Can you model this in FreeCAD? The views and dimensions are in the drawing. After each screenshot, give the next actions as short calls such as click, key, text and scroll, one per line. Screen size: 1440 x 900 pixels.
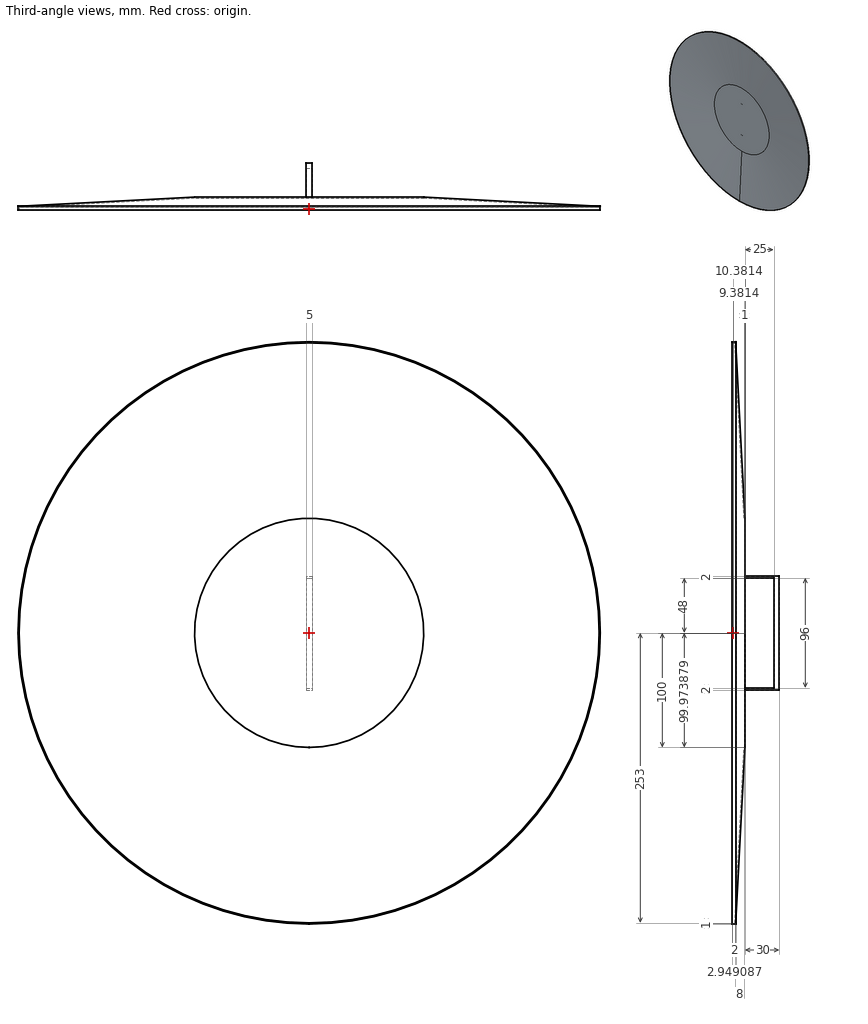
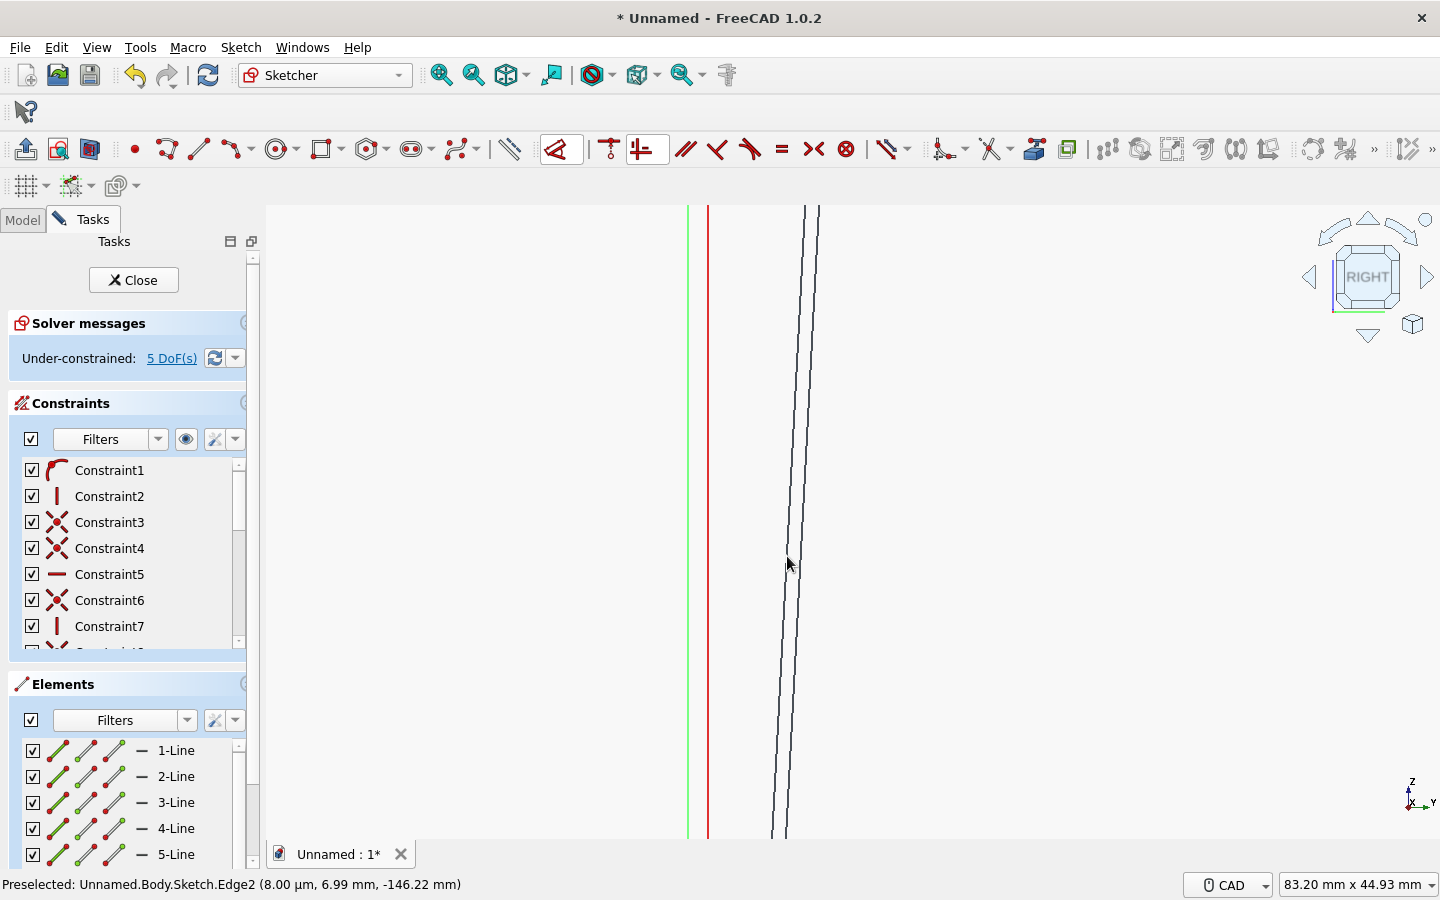
scroll(788, 551, down, 11)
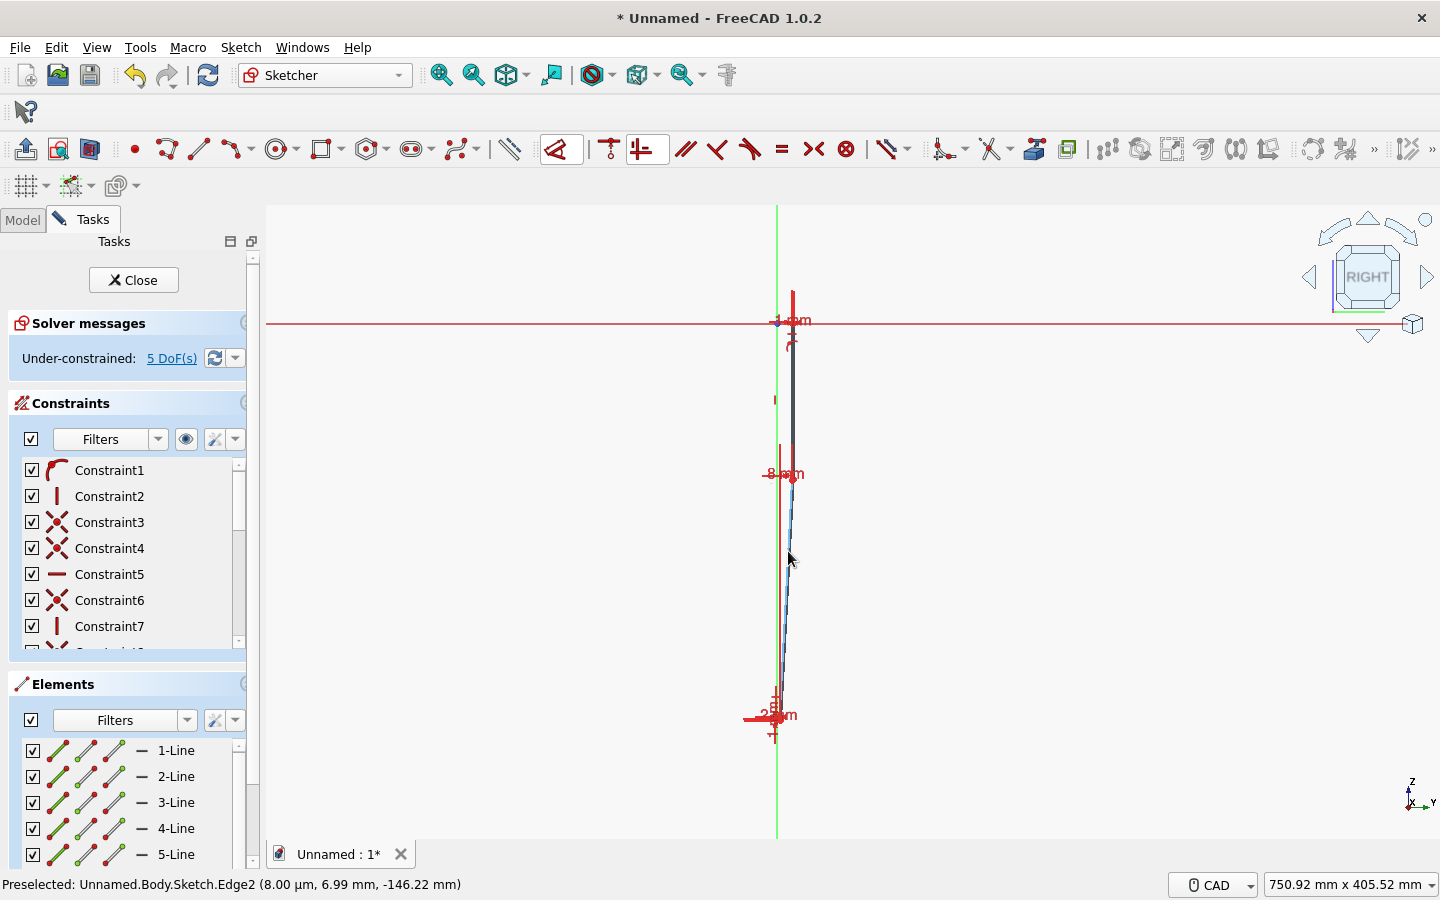
scroll(794, 433, up, 11)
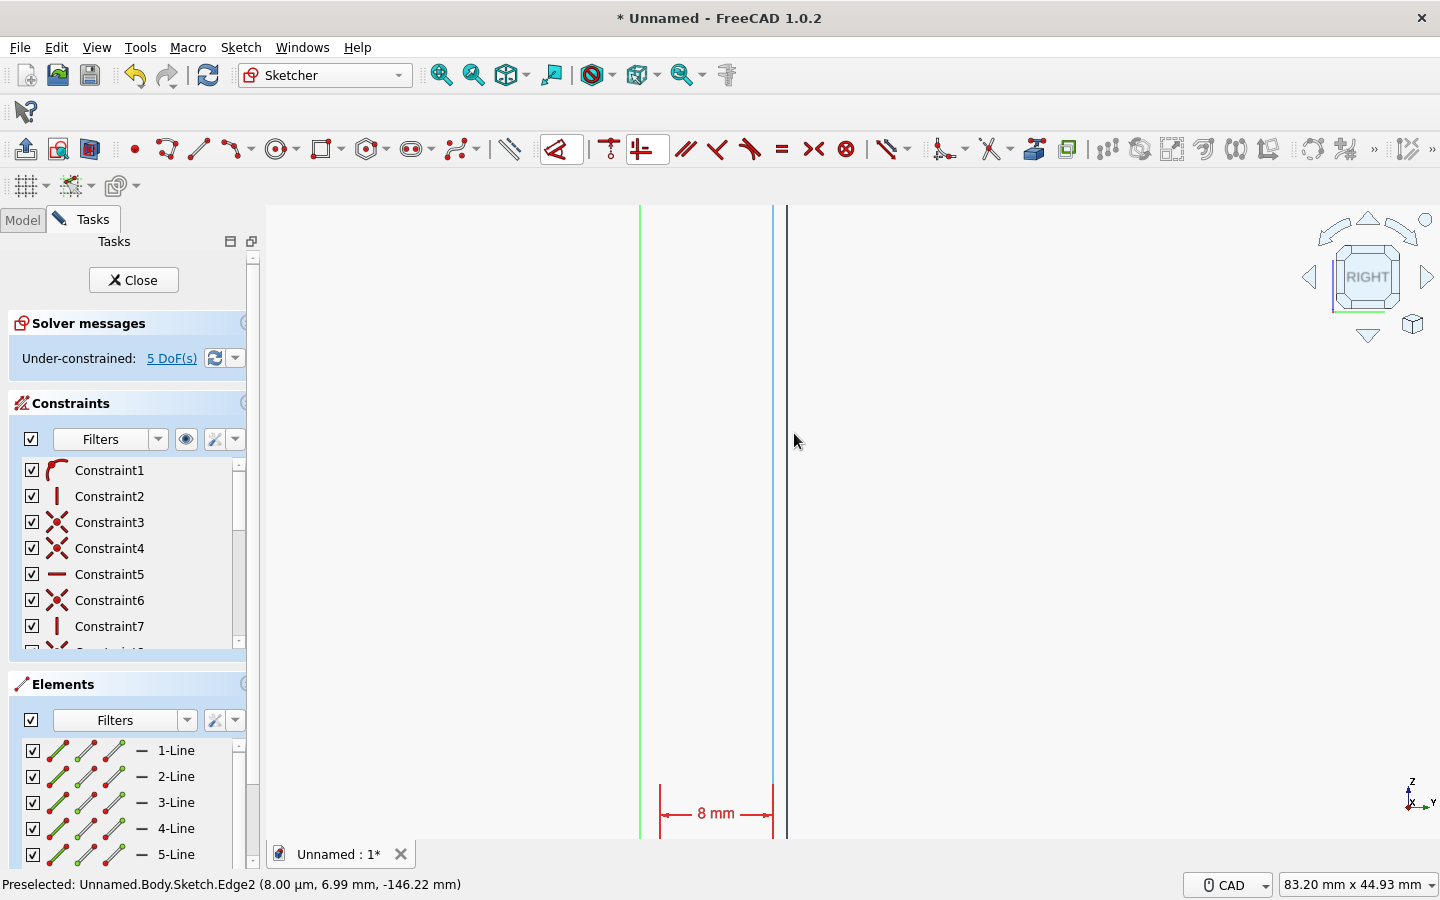
click(787, 430)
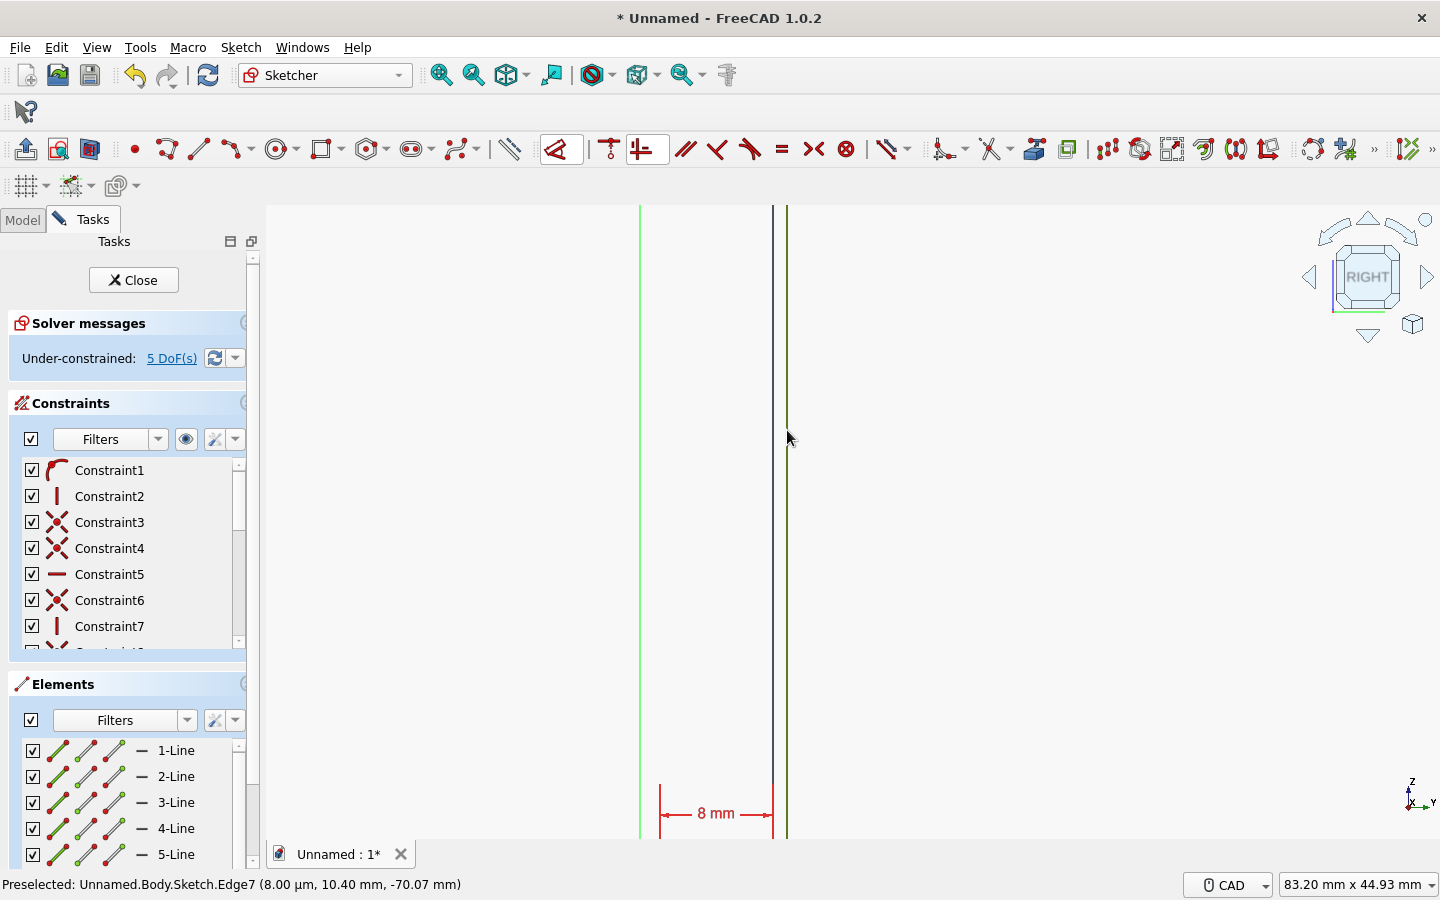
key(i)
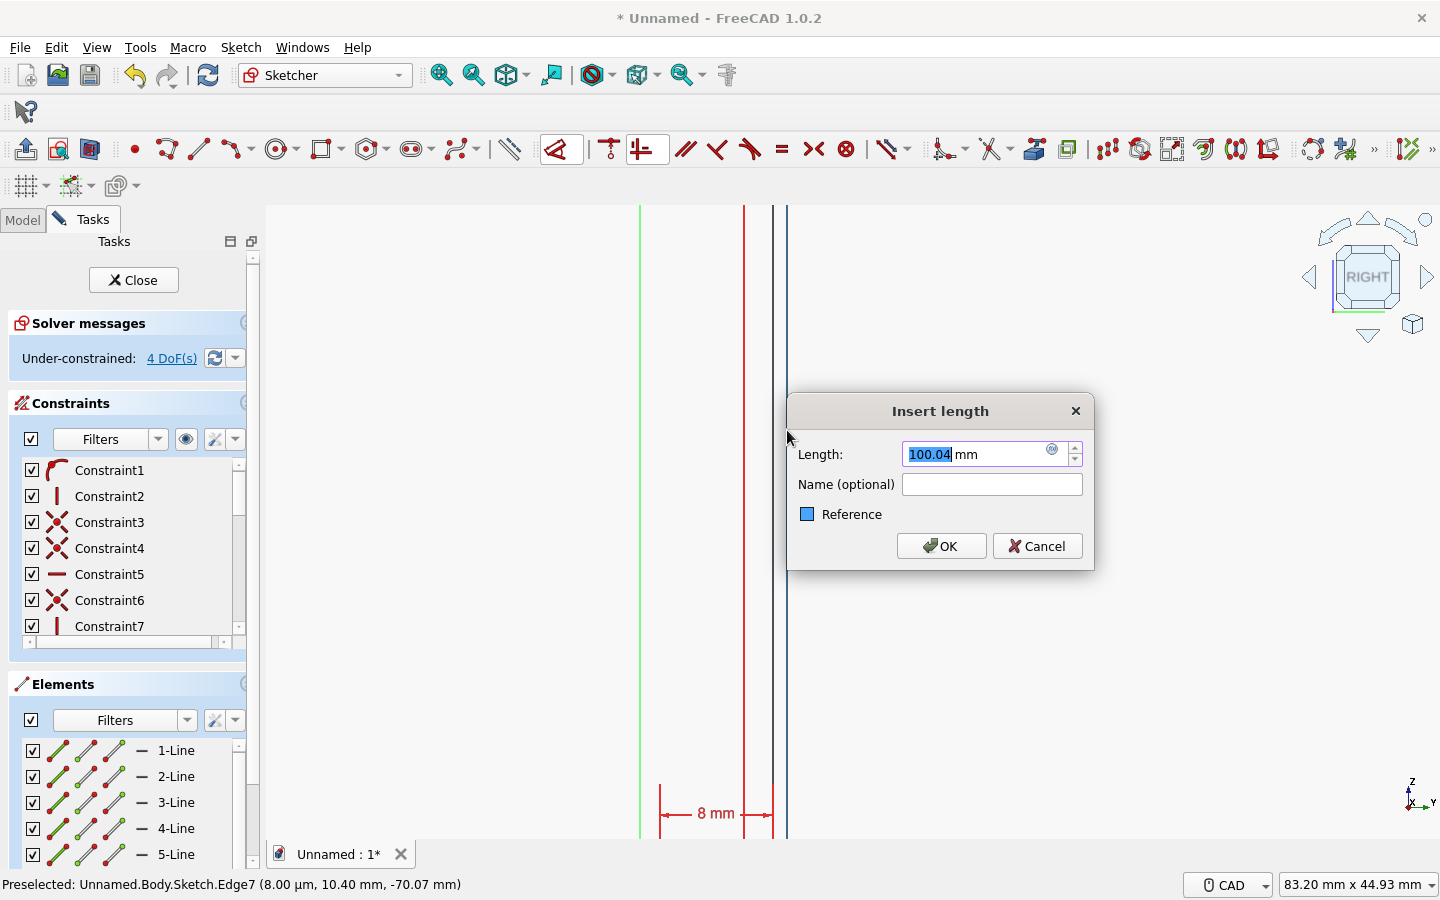
text(100)
key(Return)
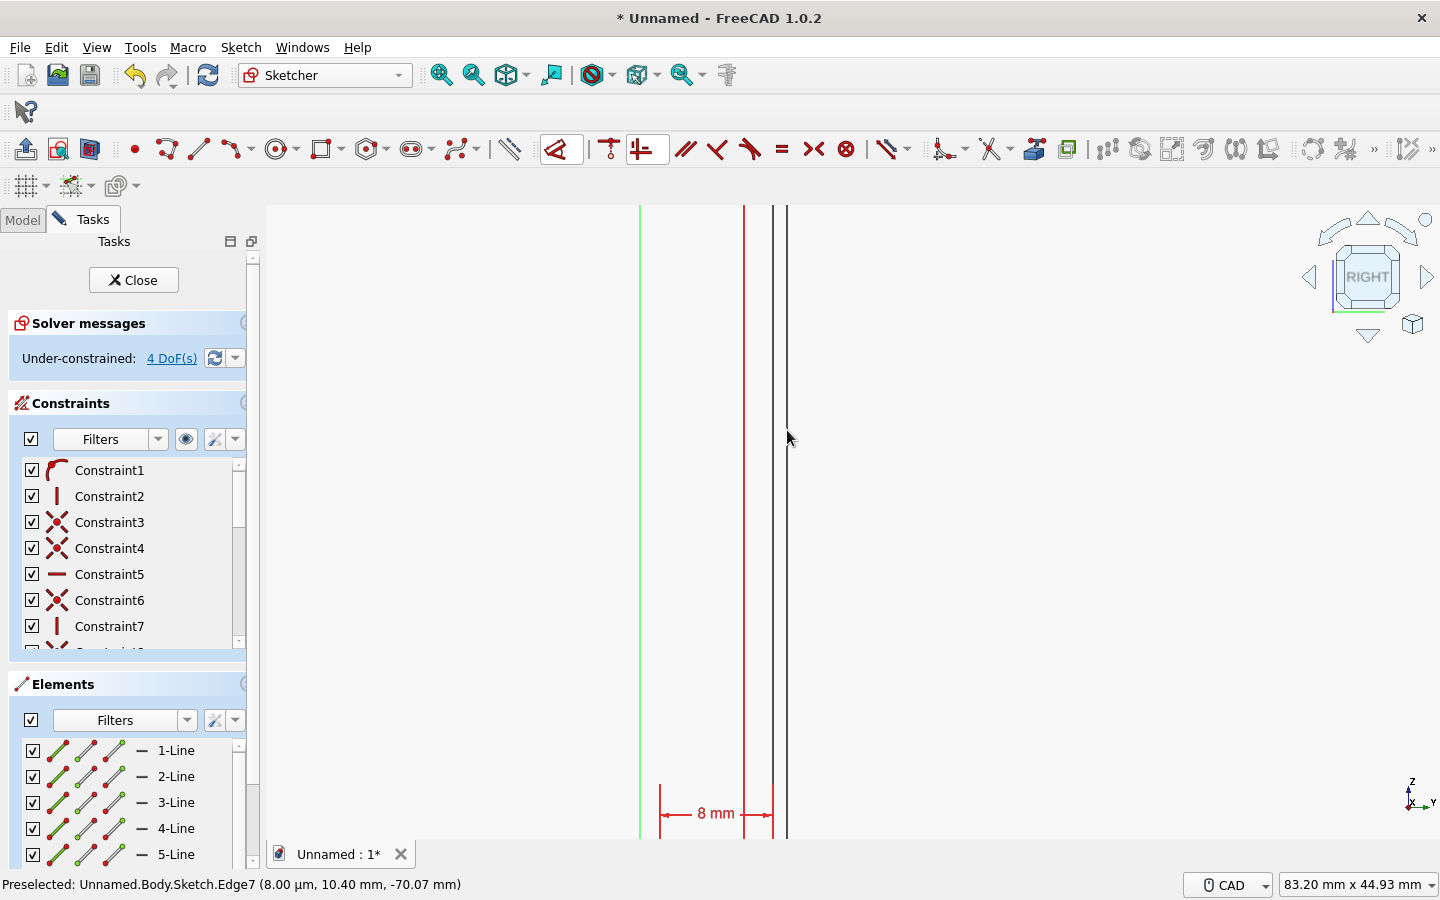
scroll(794, 433, down, 11)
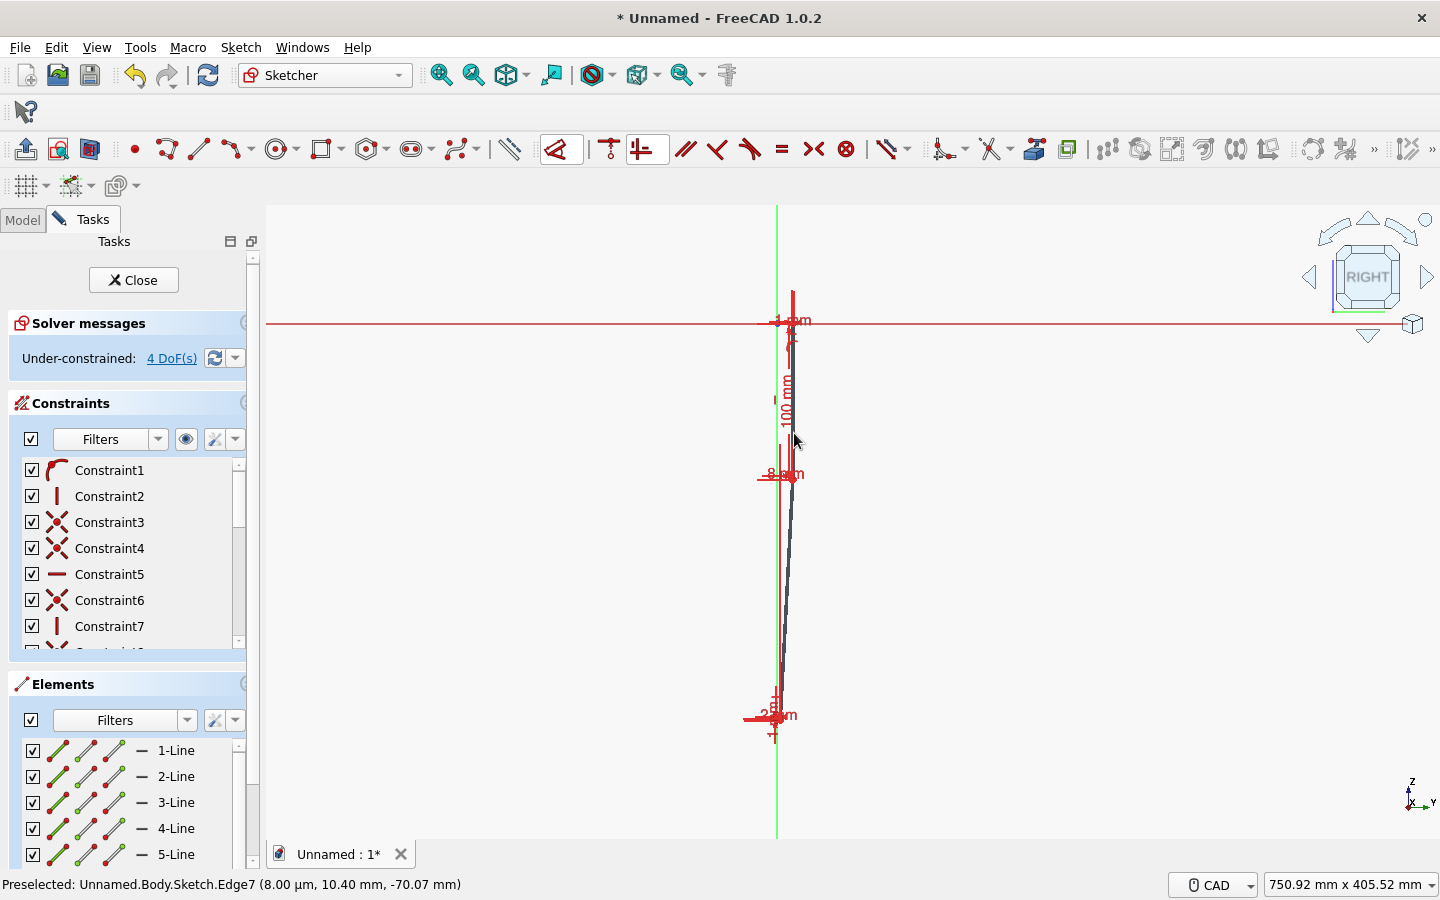
scroll(780, 719, up, 9)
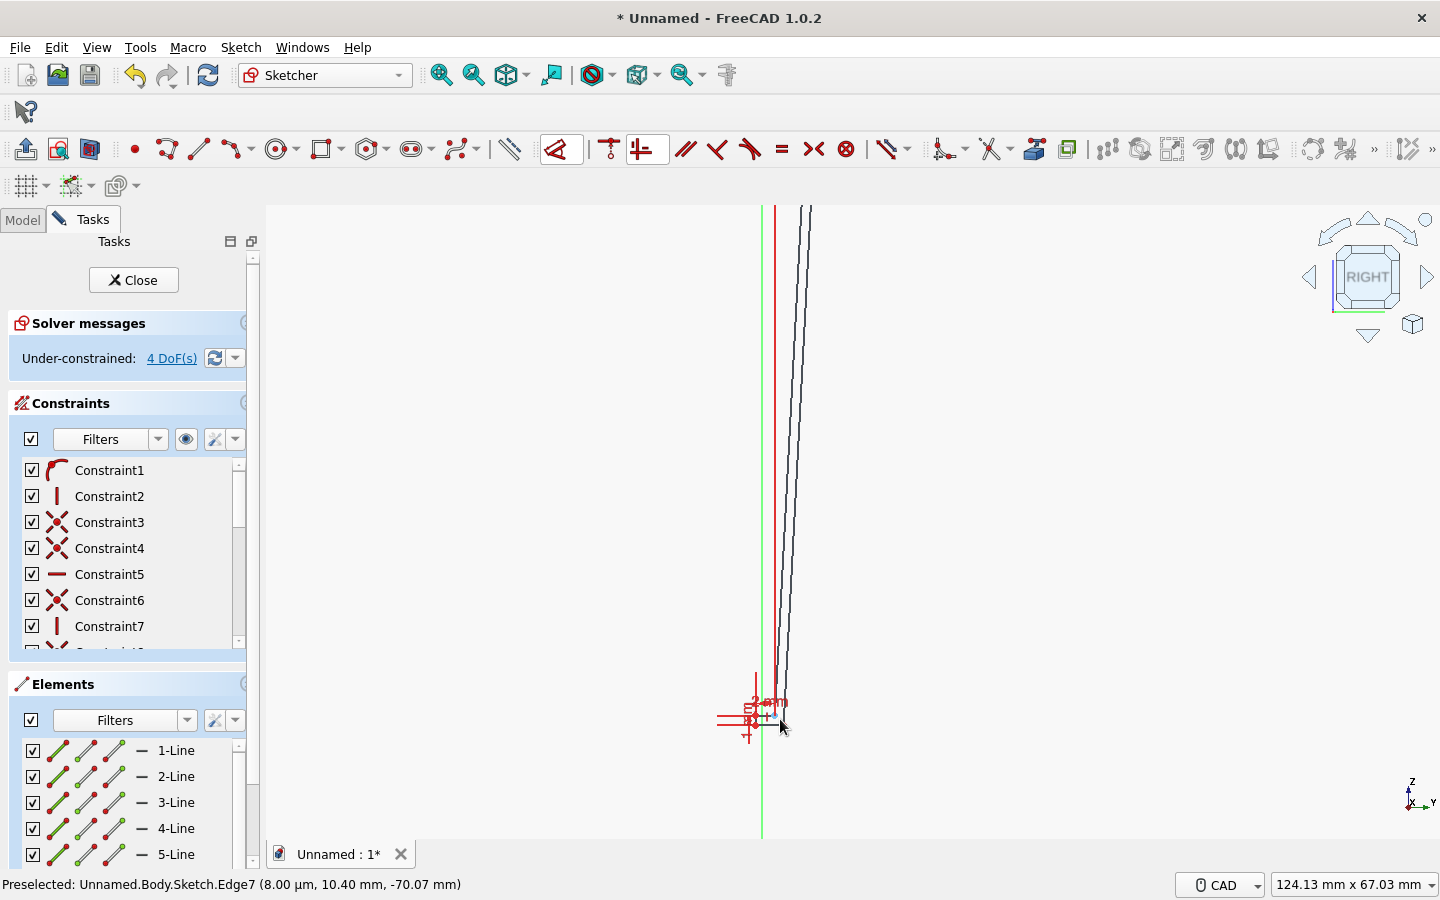
click(775, 716)